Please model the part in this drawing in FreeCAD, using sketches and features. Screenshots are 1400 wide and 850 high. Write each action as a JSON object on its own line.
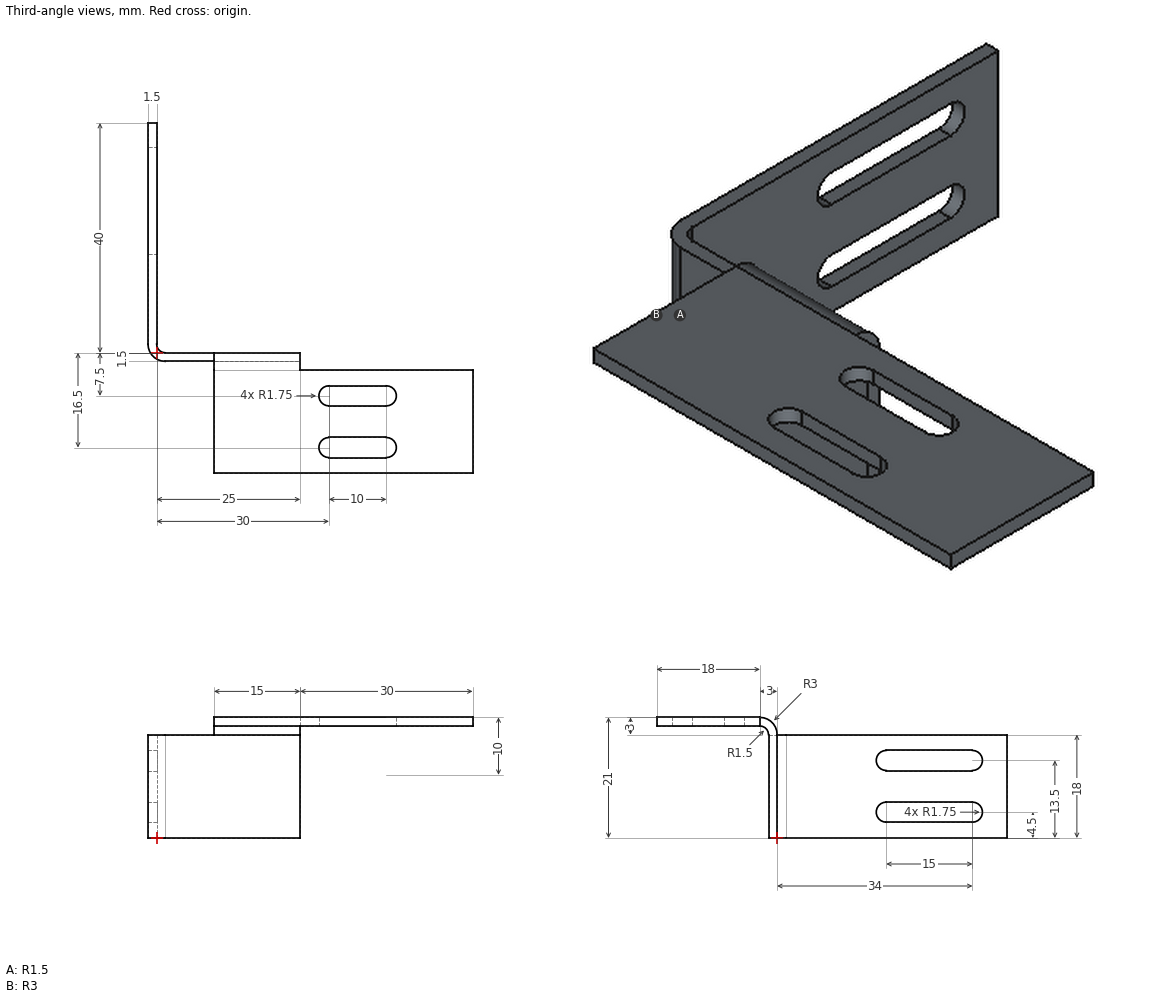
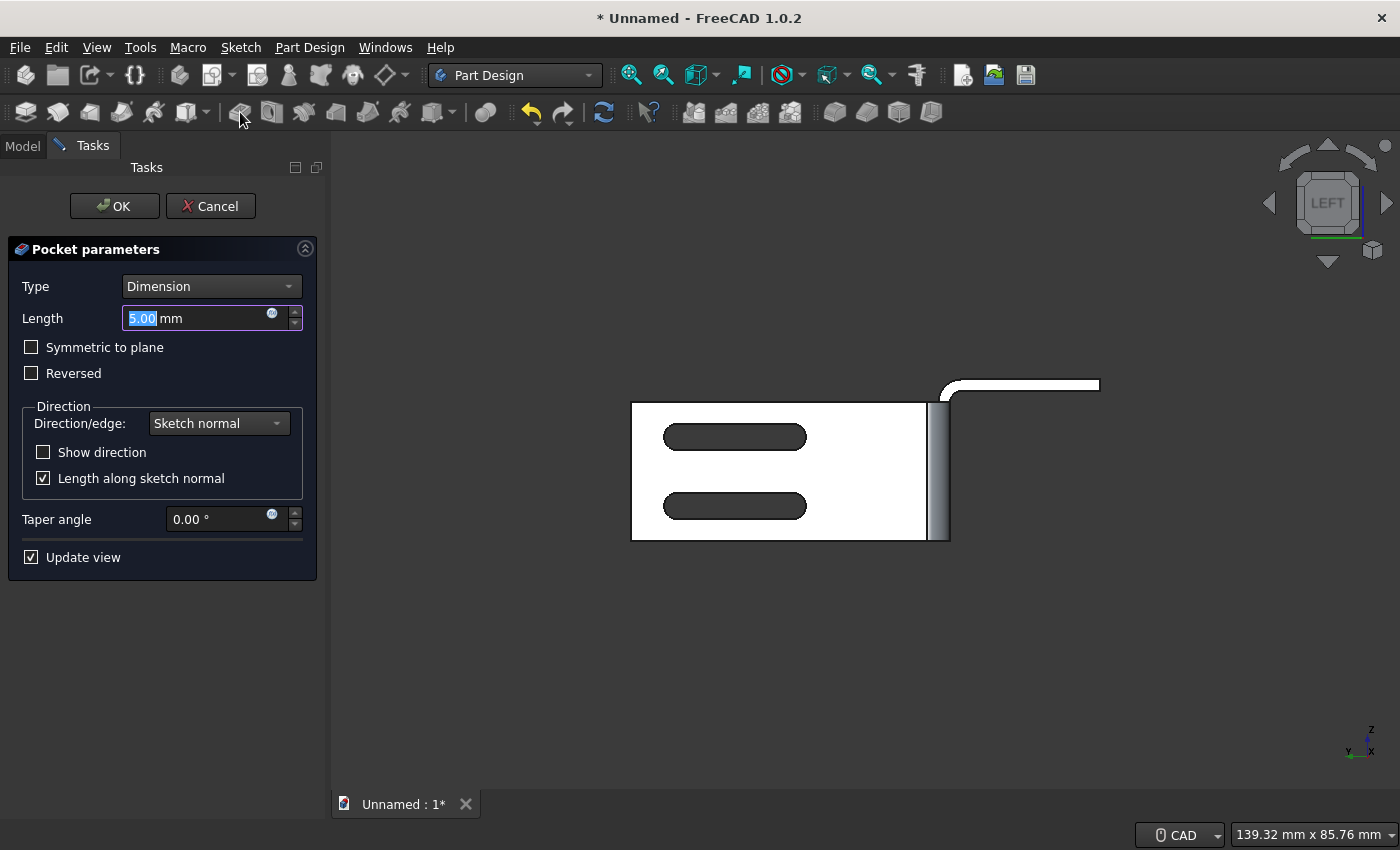
{"action": "left_click", "coordinate": [212, 286]}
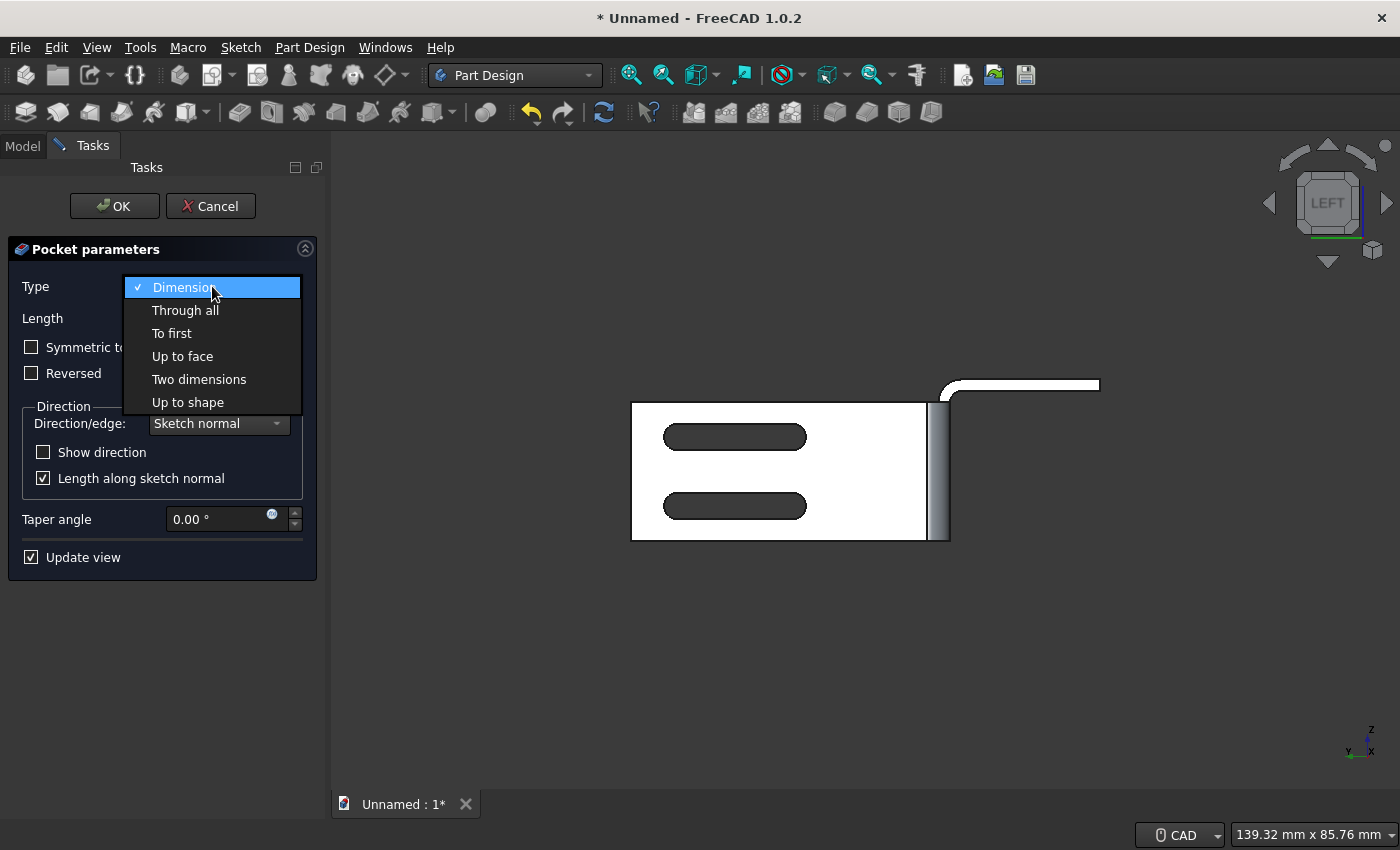
{"action": "left_click", "coordinate": [212, 310]}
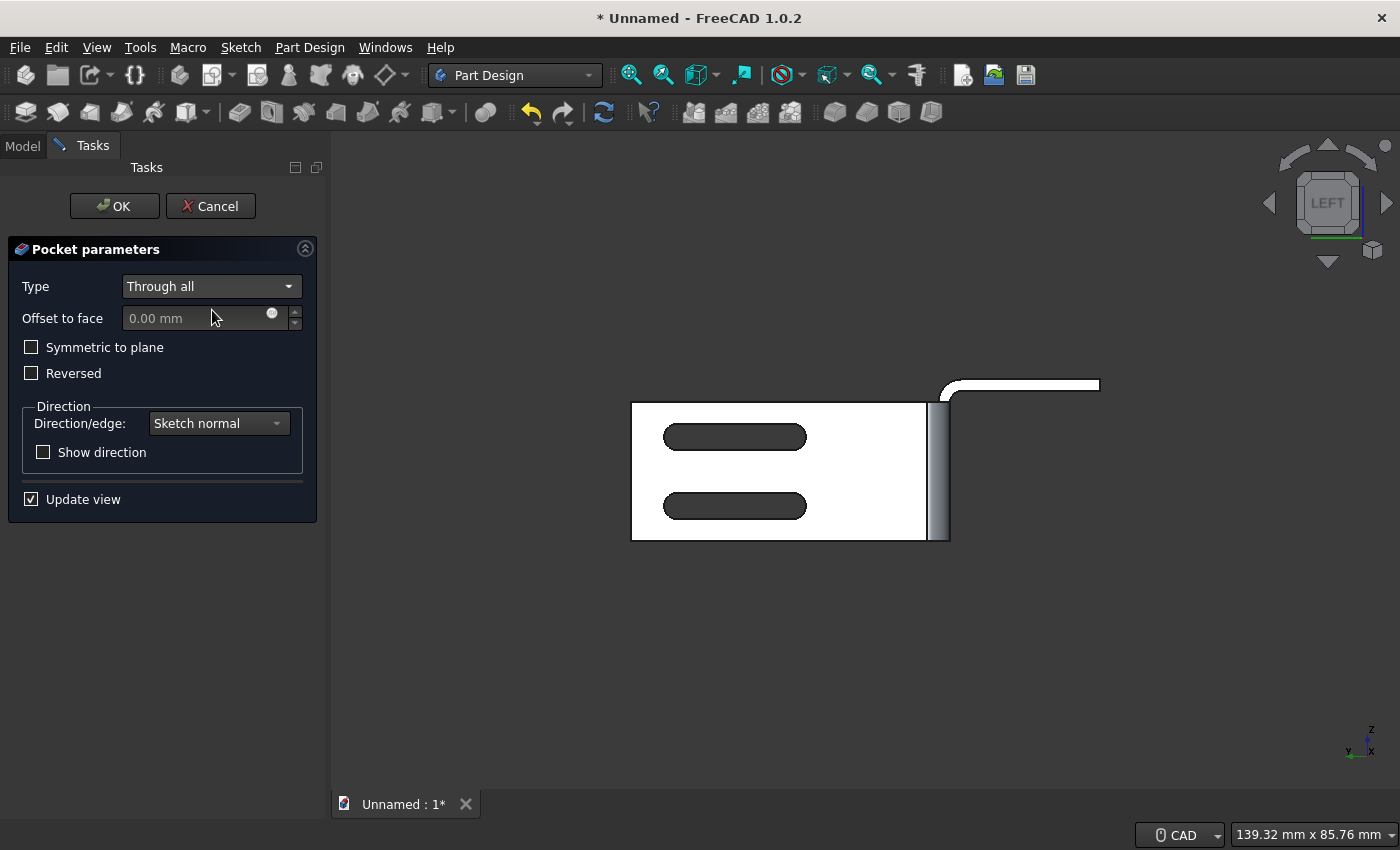
{"action": "left_click", "coordinate": [115, 206]}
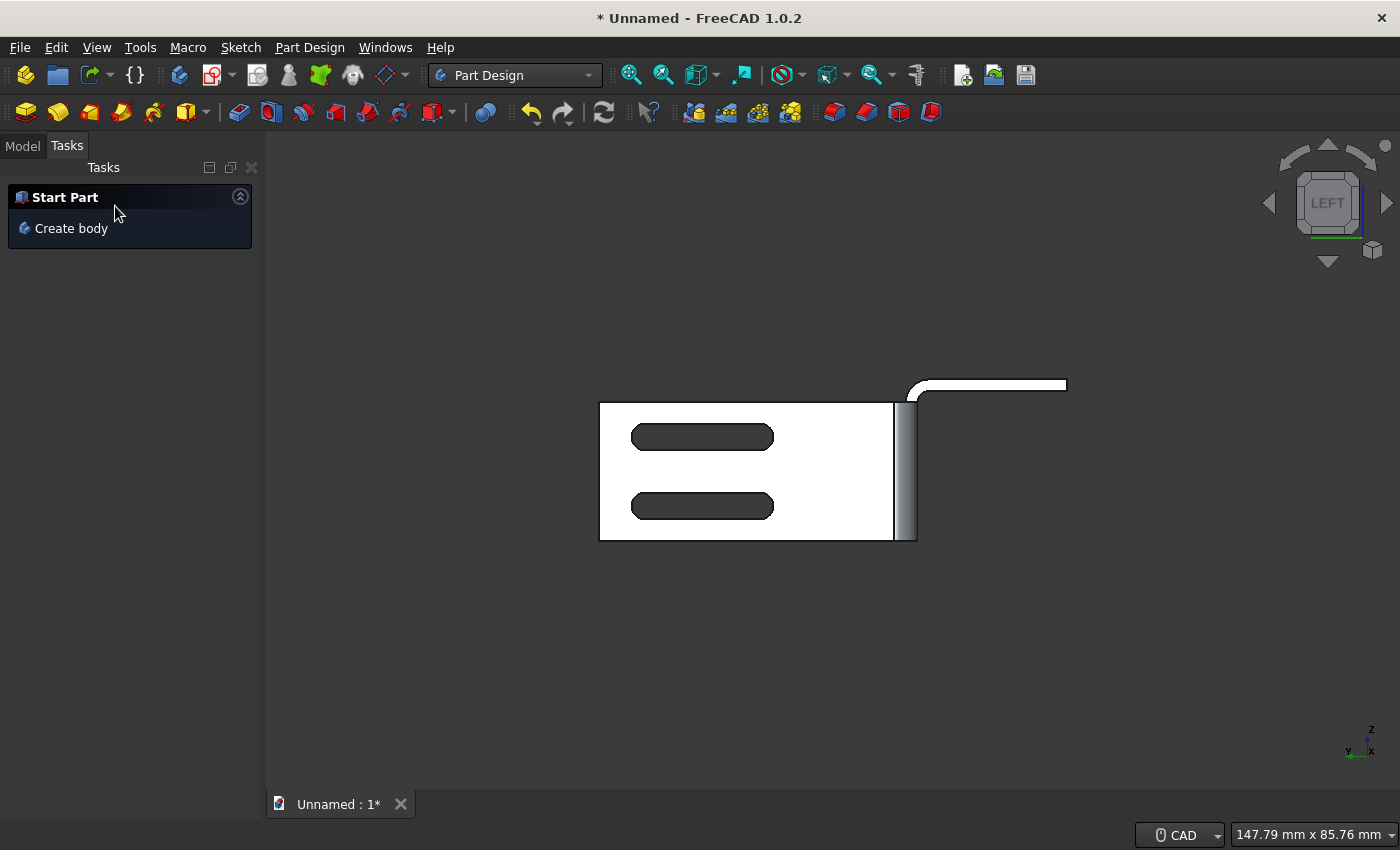
{"action": "left_click", "coordinate": [632, 76]}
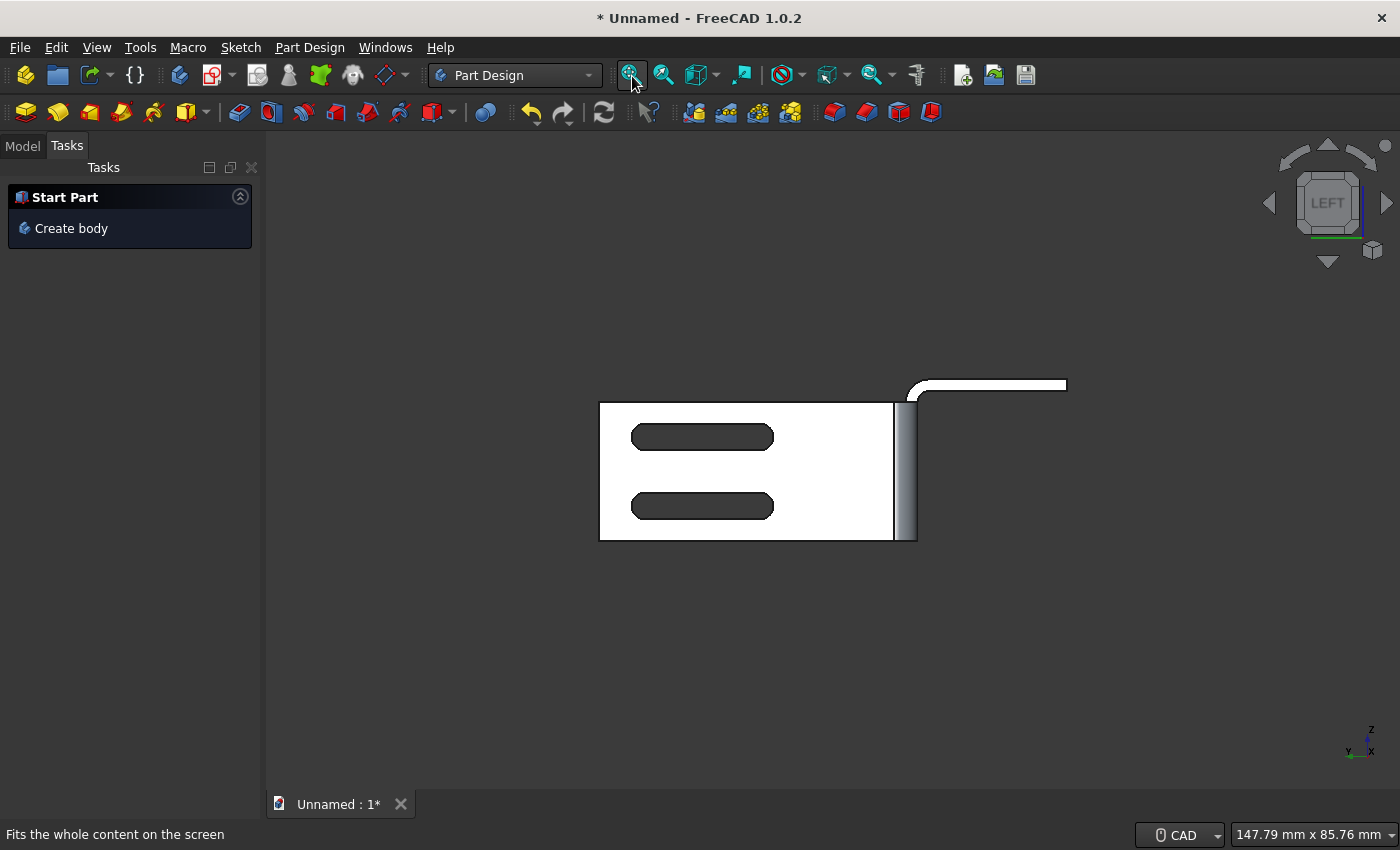
{"action": "key", "text": "0"}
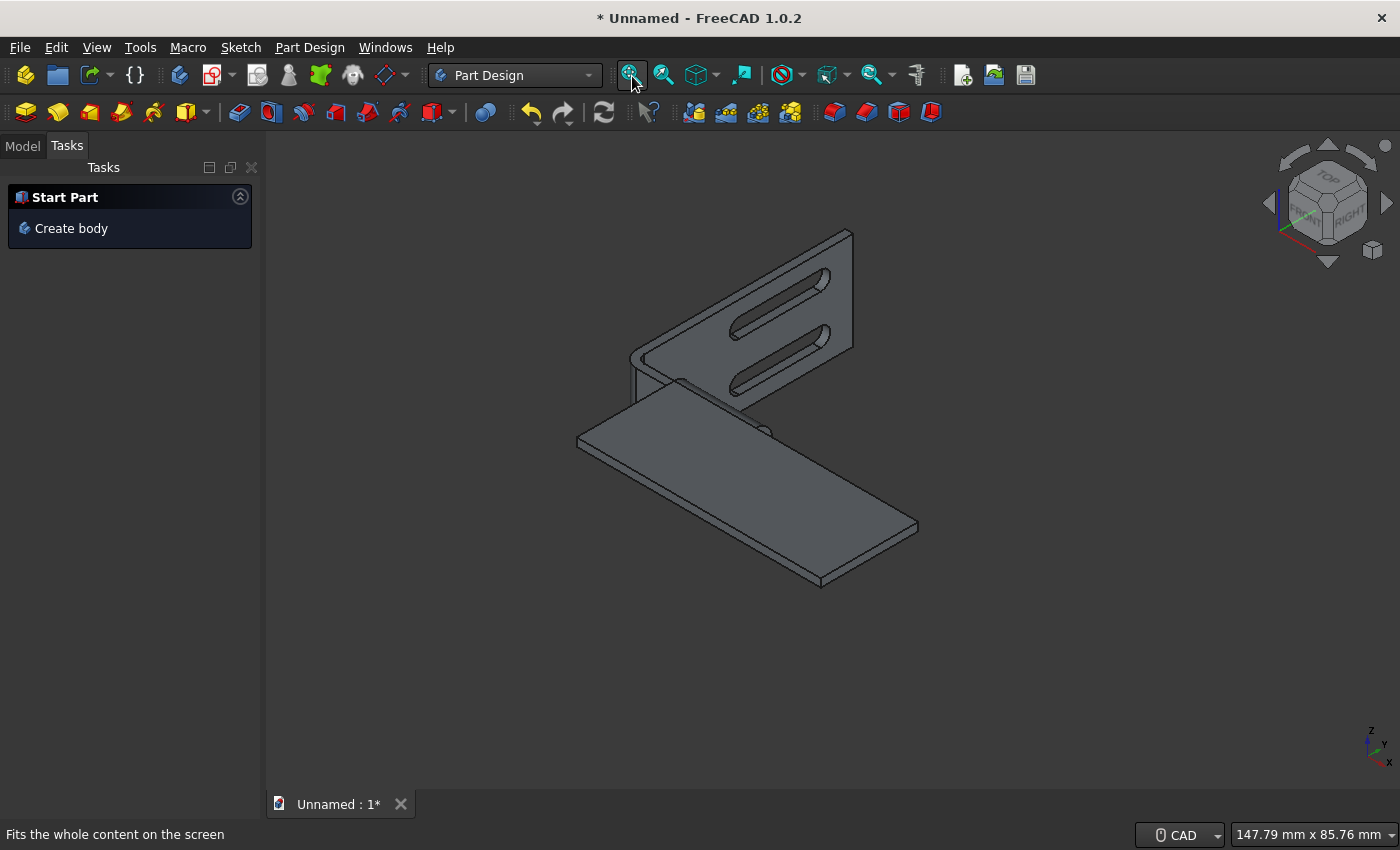
{"action": "left_click", "coordinate": [817, 519]}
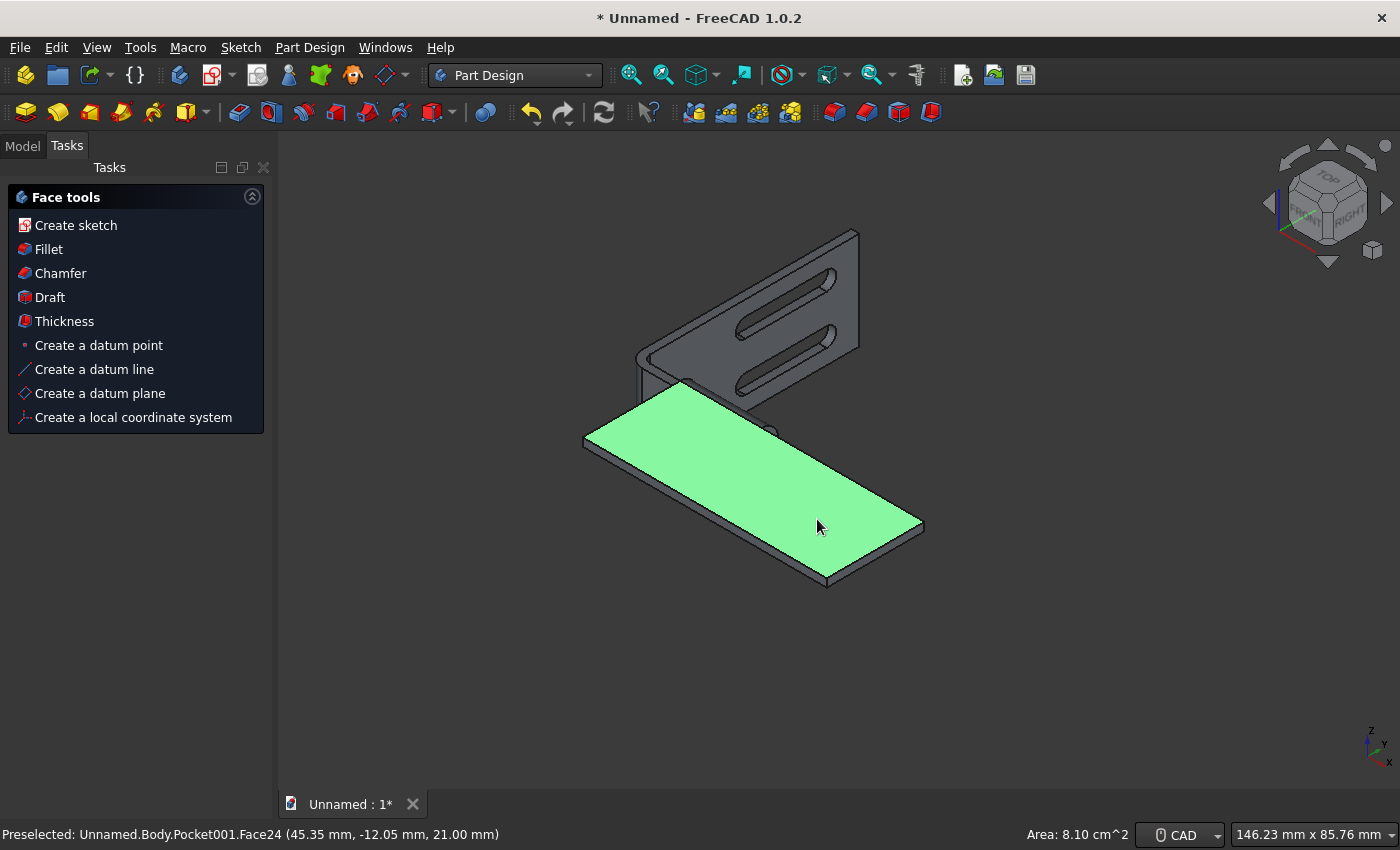
{"action": "left_click", "coordinate": [212, 76]}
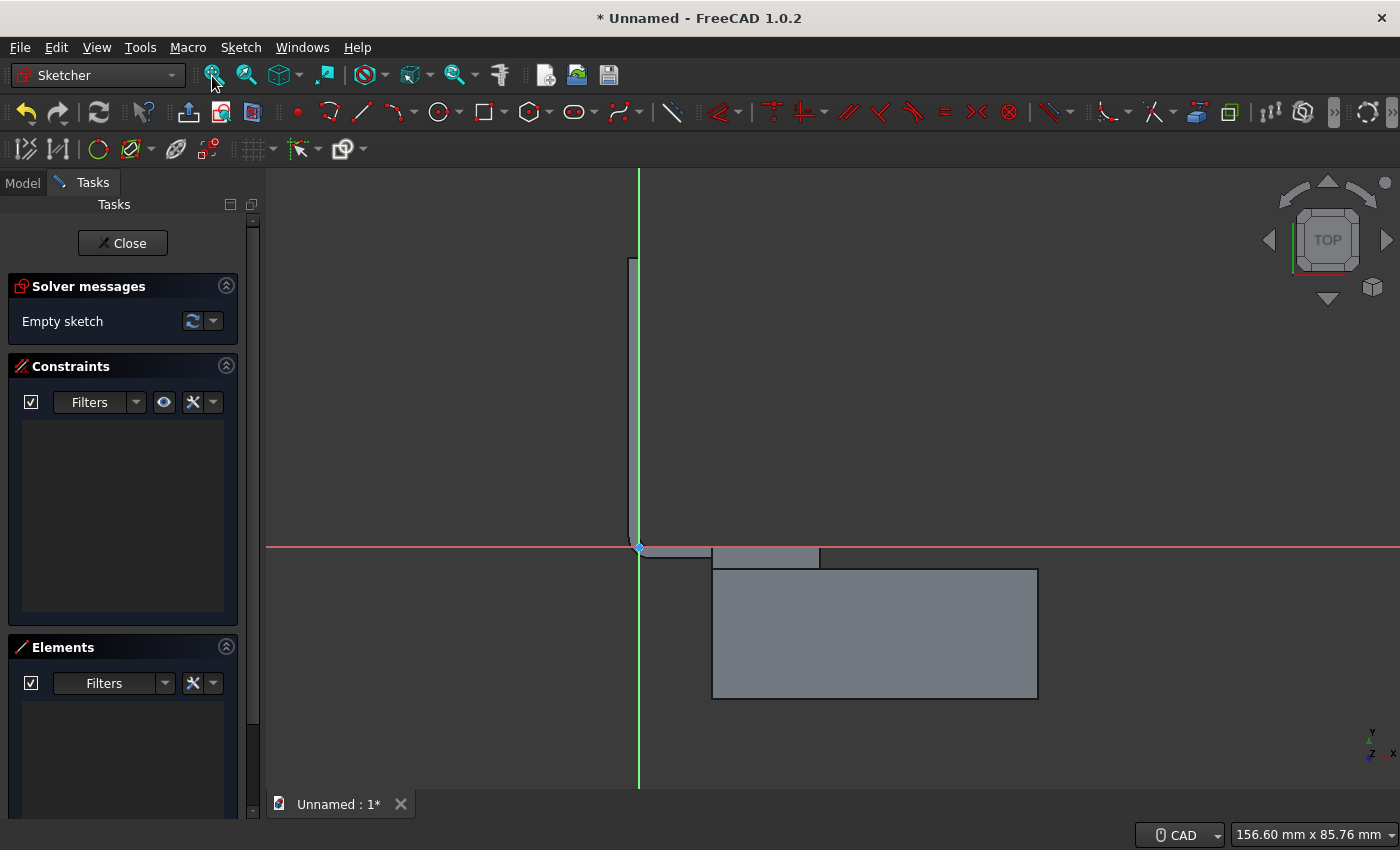
{"action": "scroll", "coordinate": [935, 685], "scroll_direction": "up", "scroll_amount": 7}